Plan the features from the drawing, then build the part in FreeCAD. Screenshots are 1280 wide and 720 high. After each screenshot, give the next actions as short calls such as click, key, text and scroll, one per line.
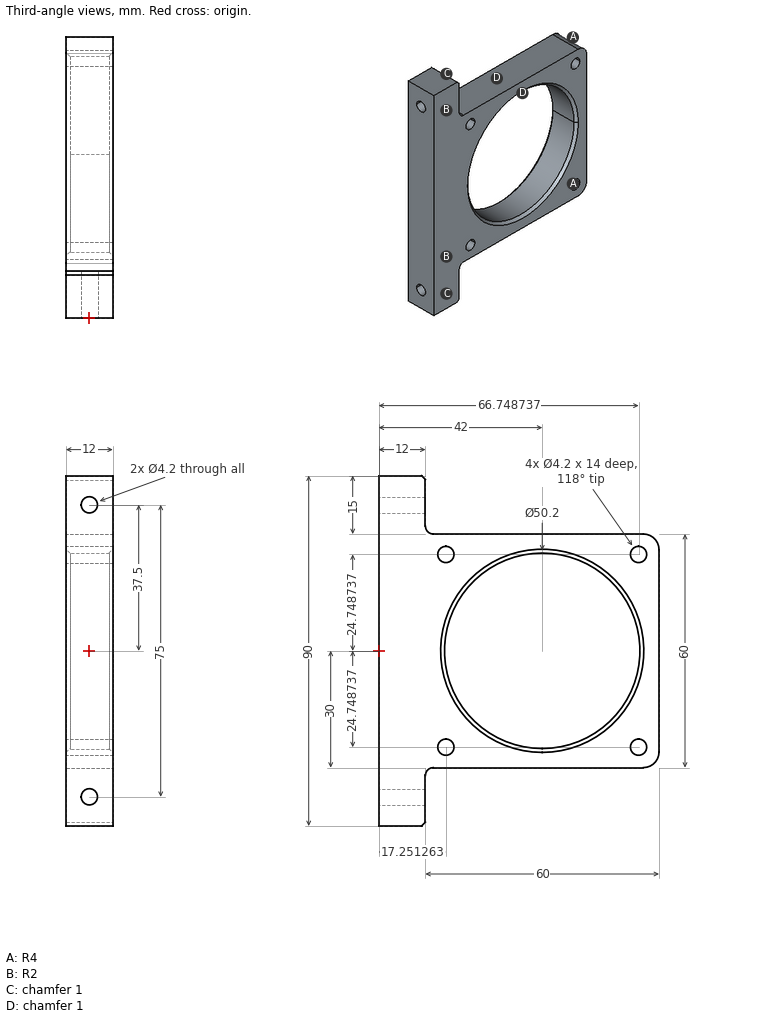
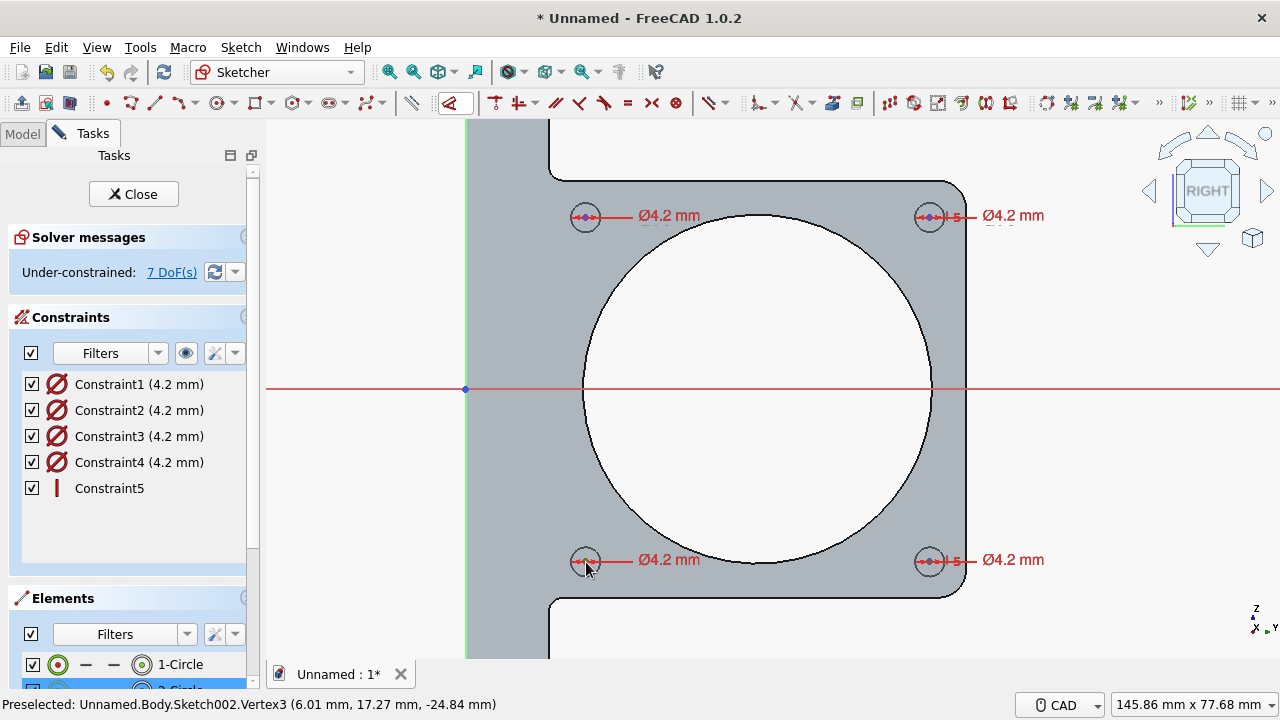
click(538, 104)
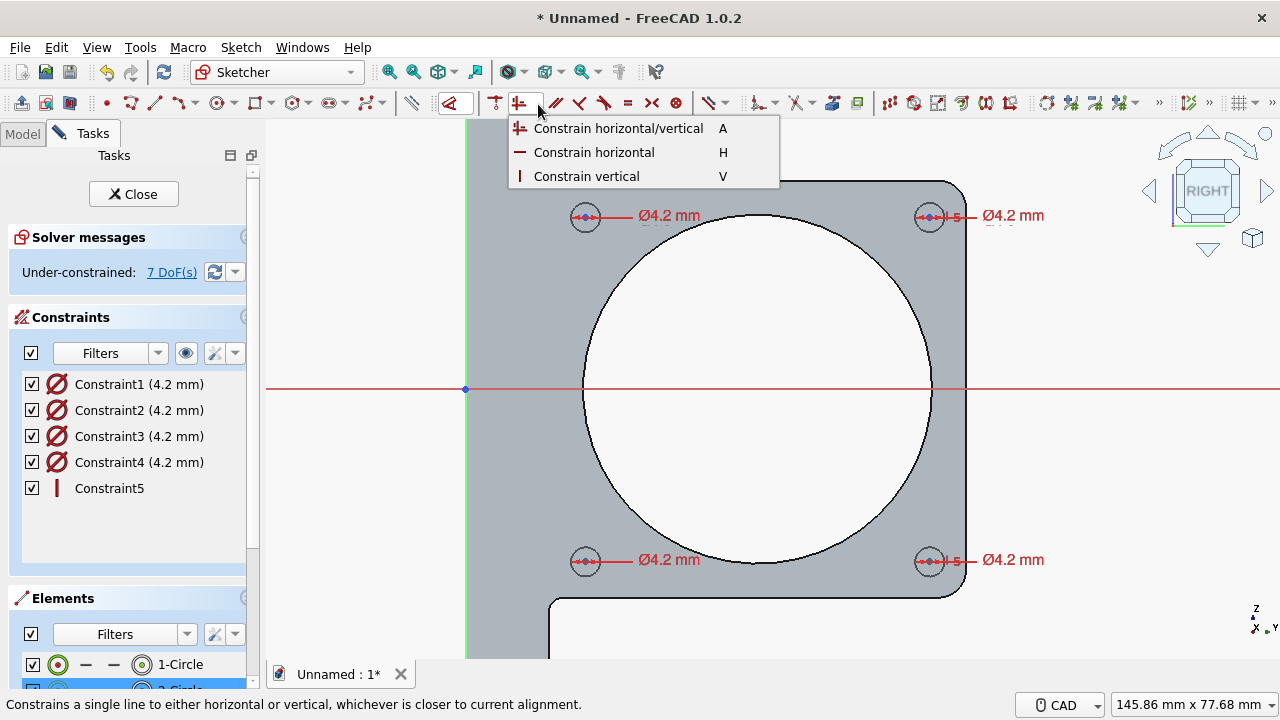
click(644, 152)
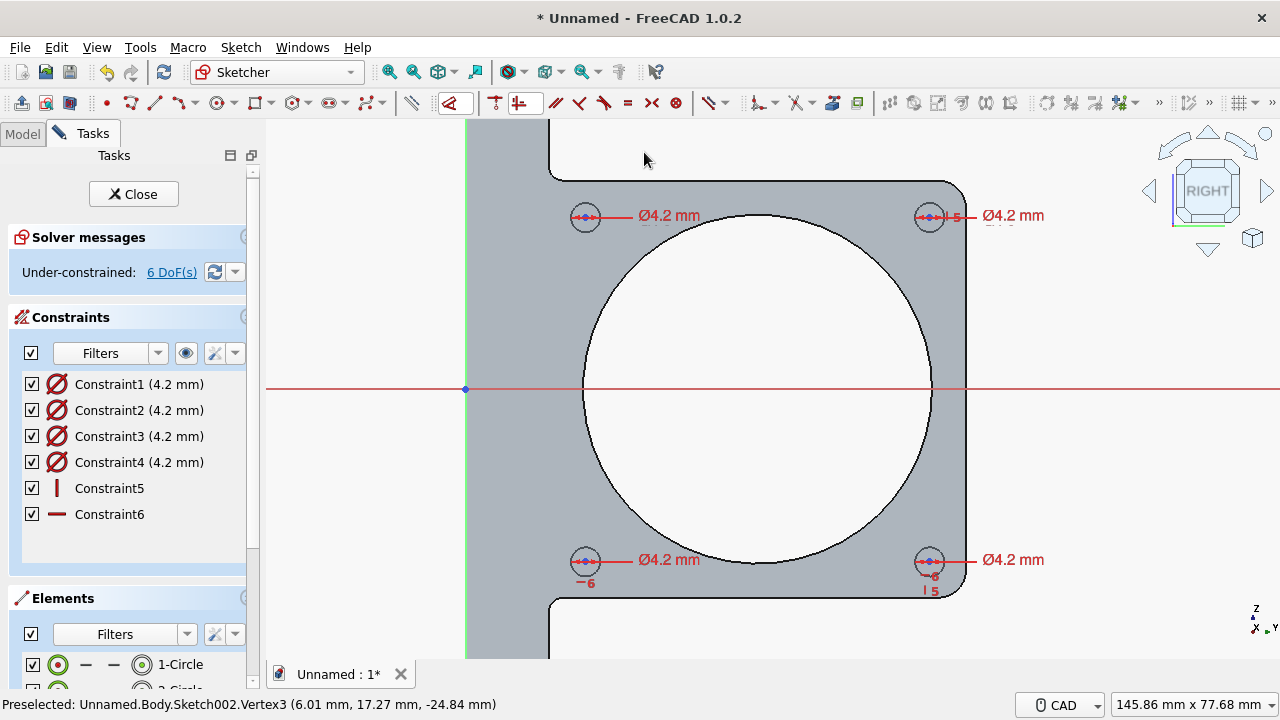
click(586, 562)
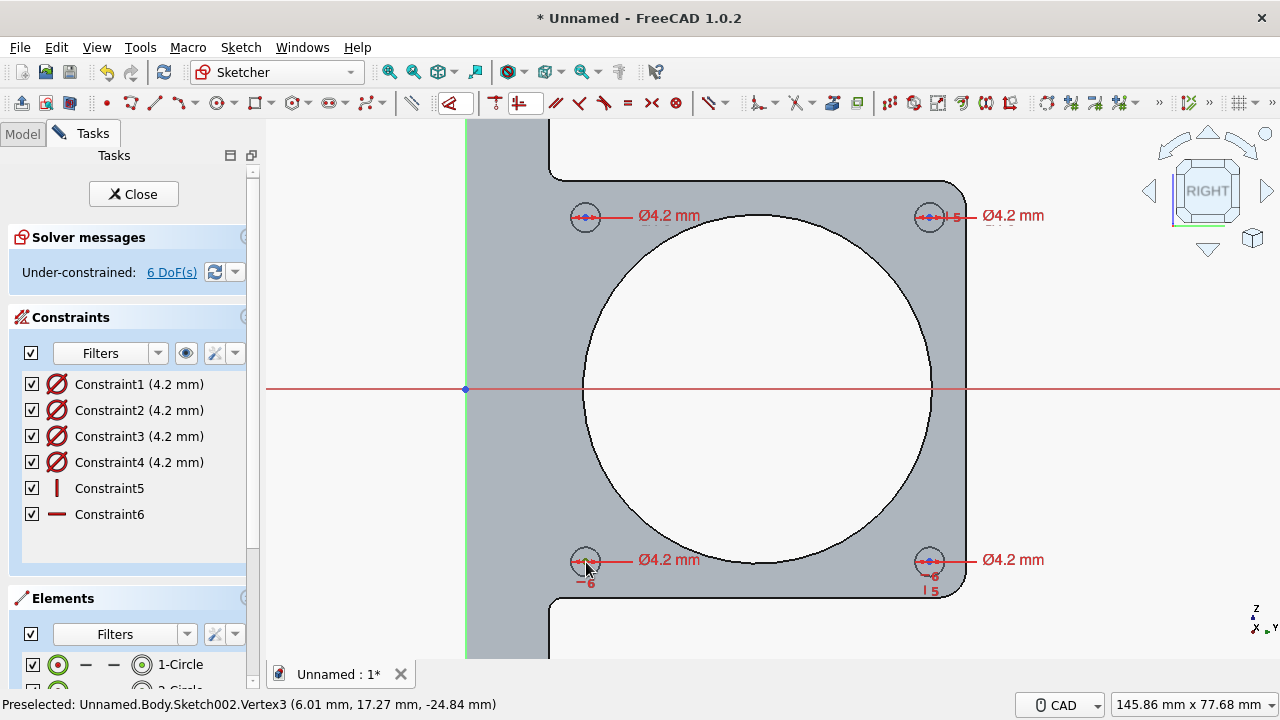
click(586, 218)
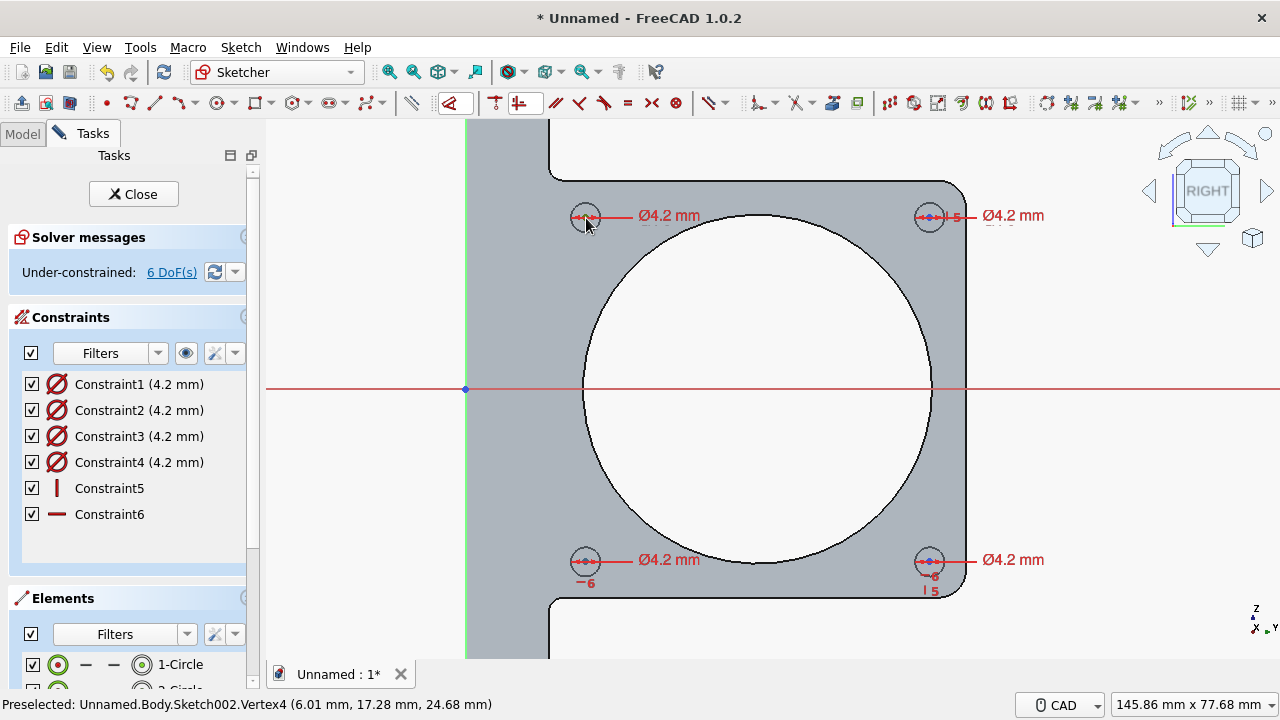
click(538, 104)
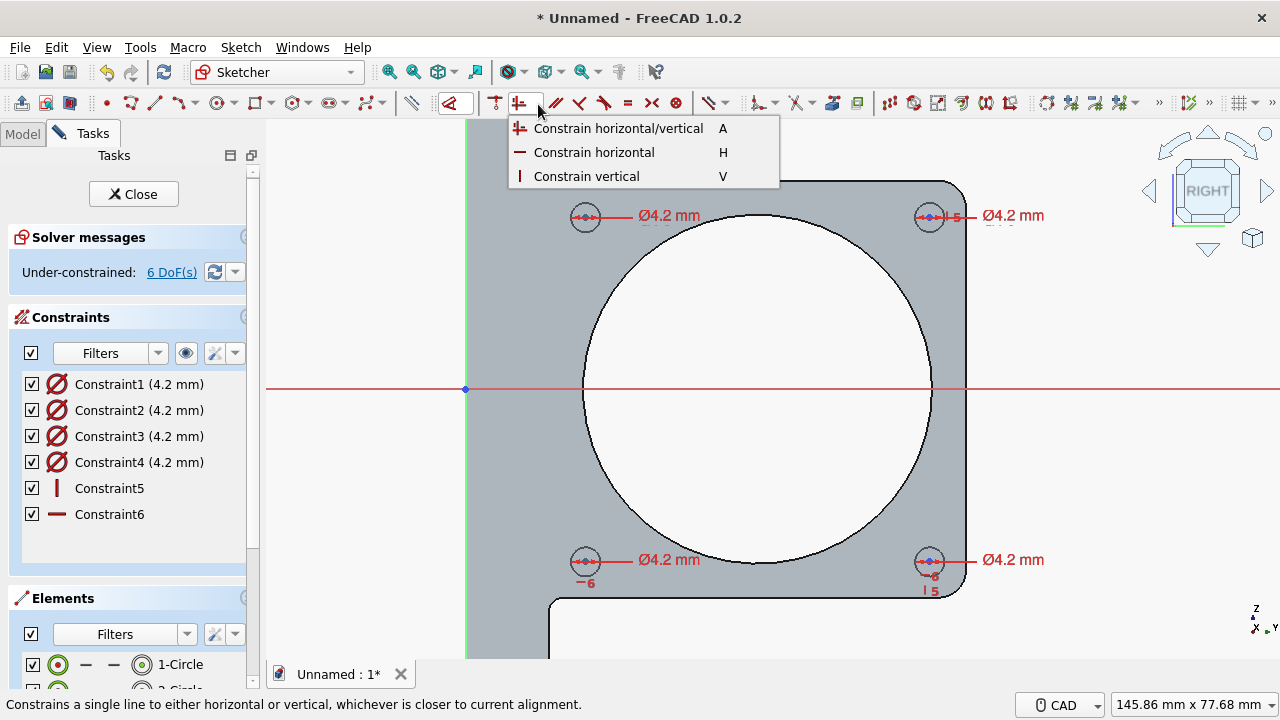
click(644, 176)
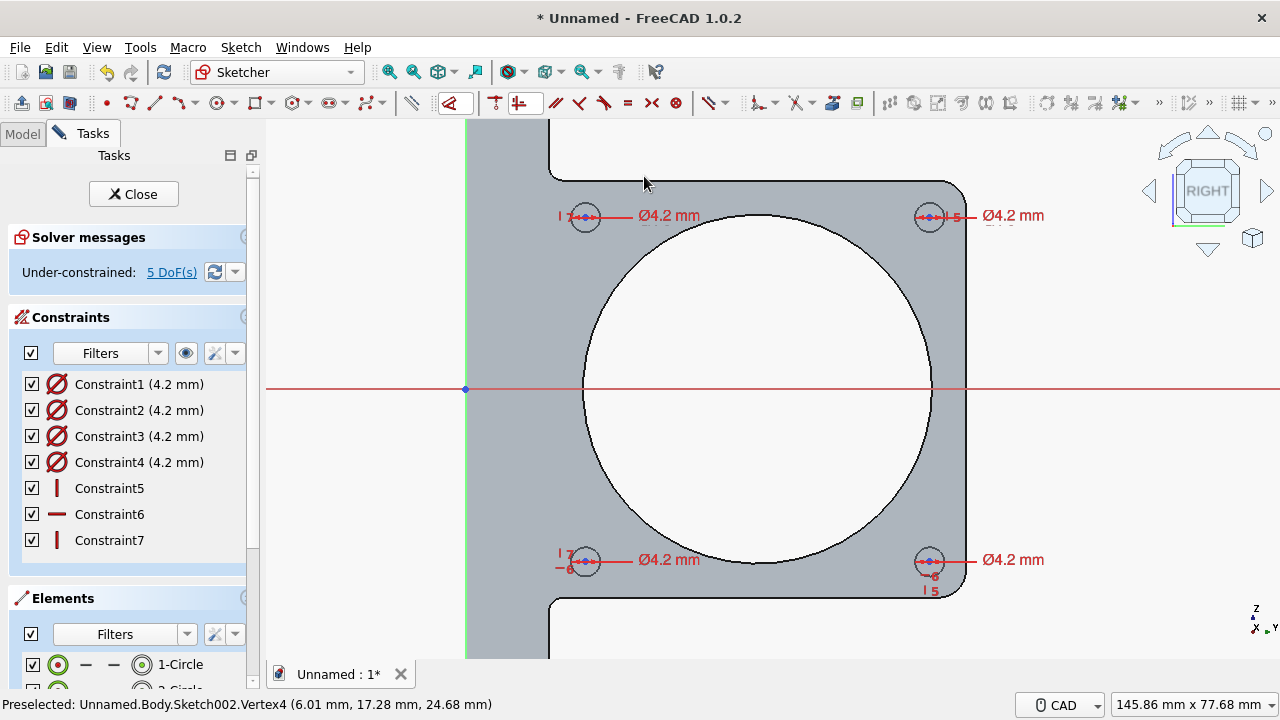
click(930, 218)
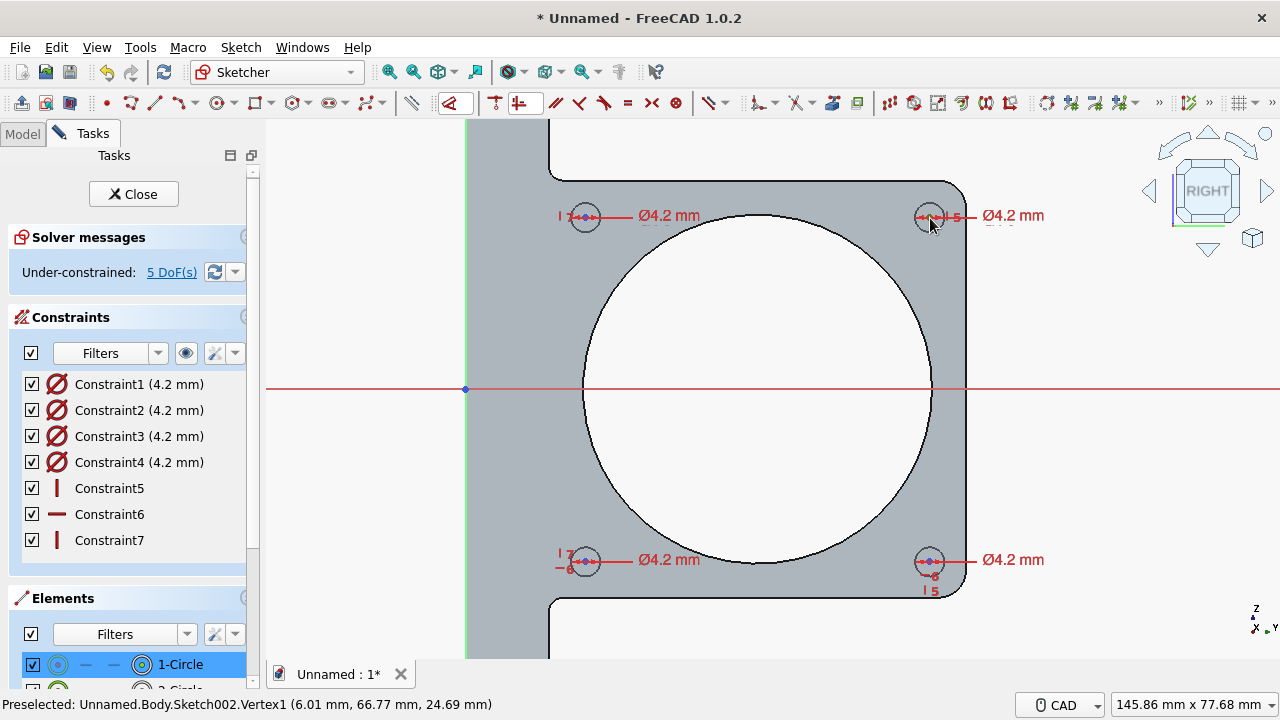
click(586, 218)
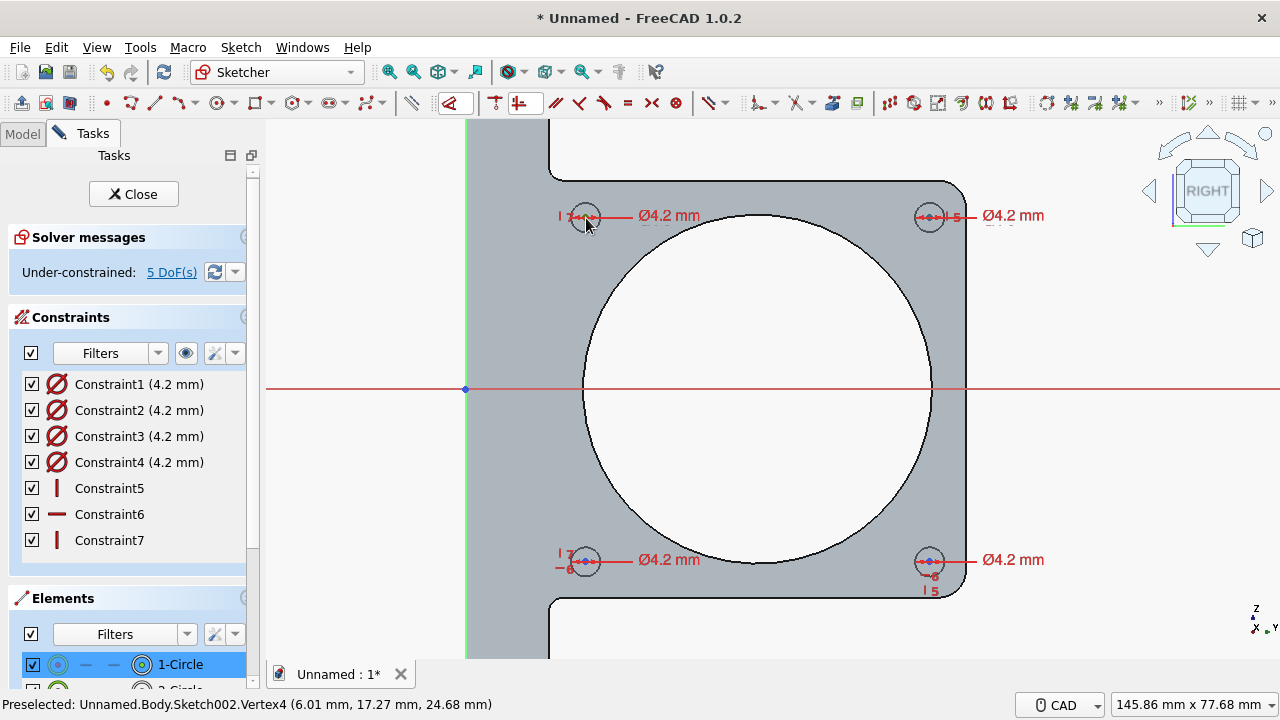
key(h)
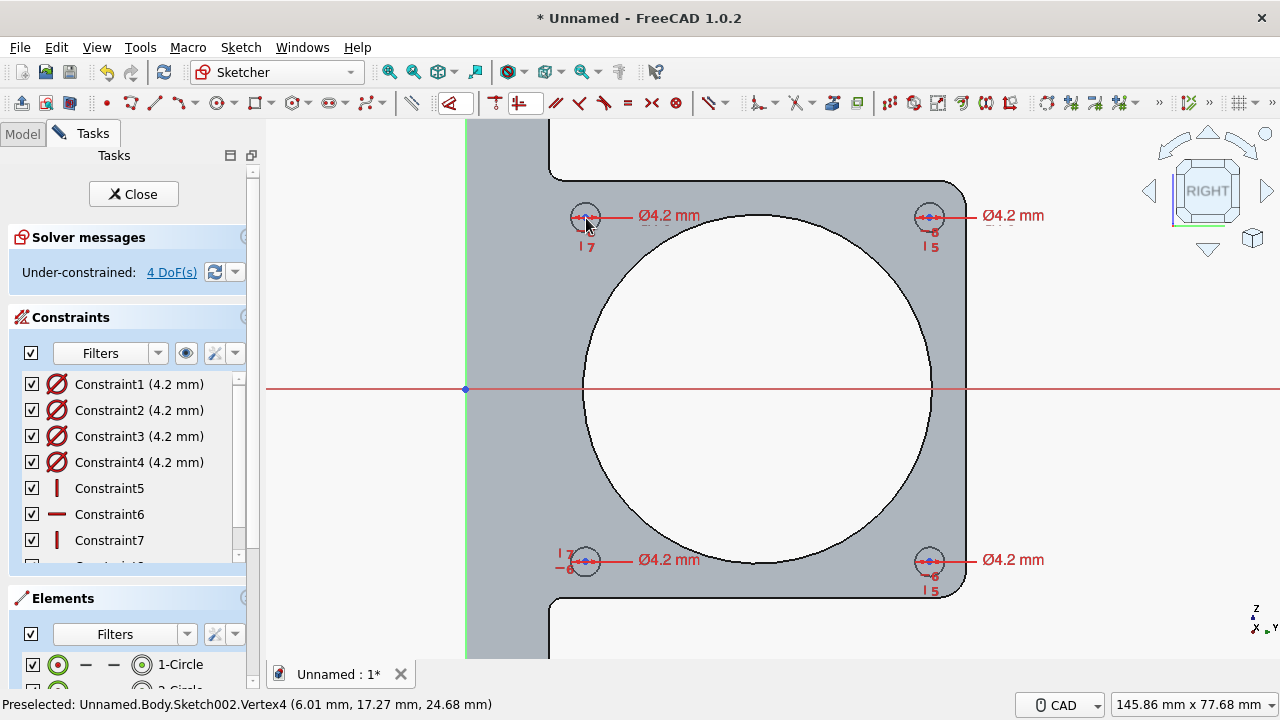
click(930, 218)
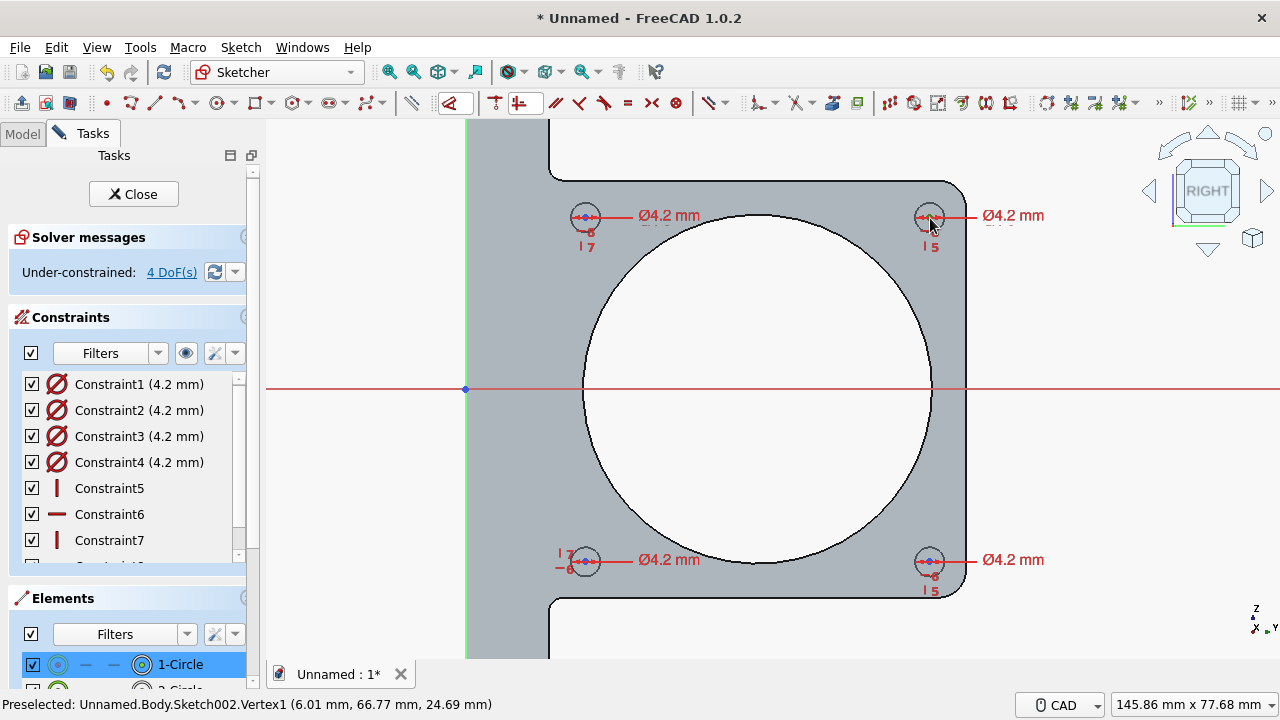
key(l)